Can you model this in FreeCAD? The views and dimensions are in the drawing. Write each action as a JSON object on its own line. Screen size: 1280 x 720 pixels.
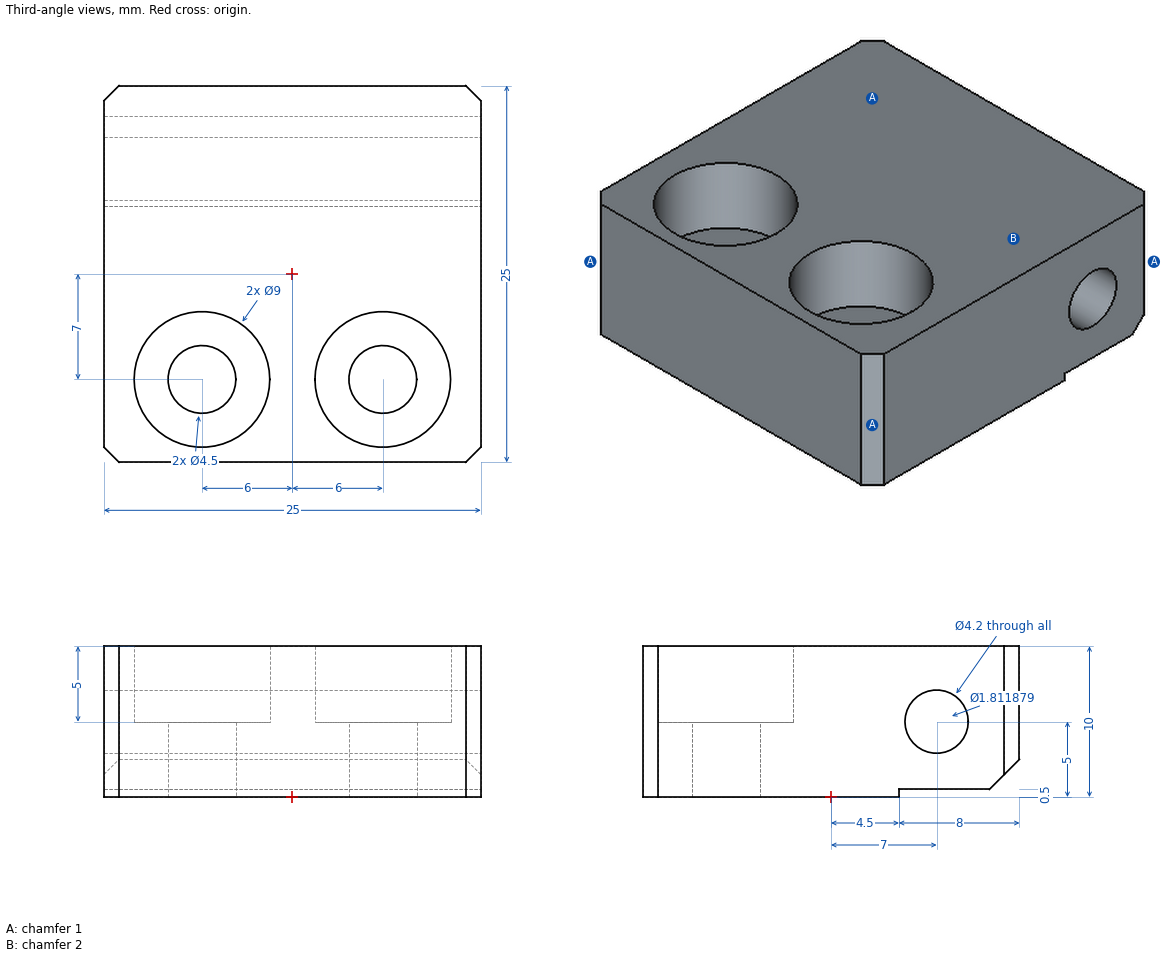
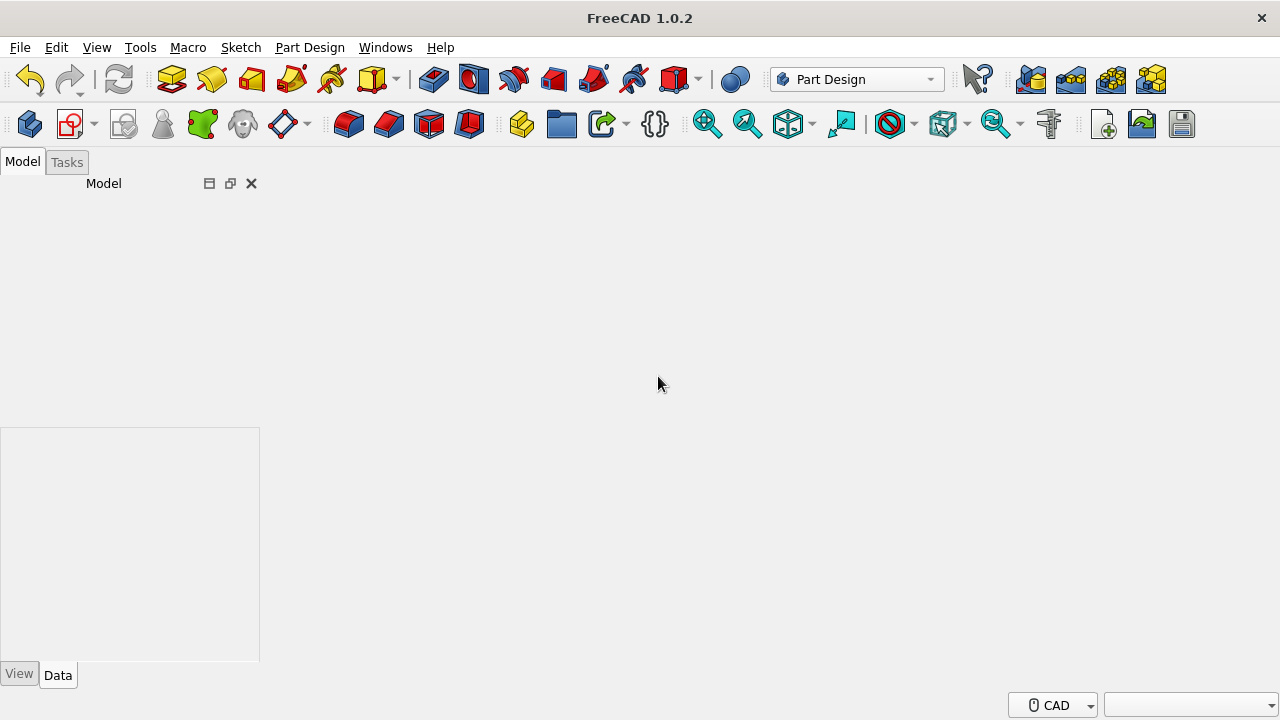
{"action": "key", "text": "ctrl+n"}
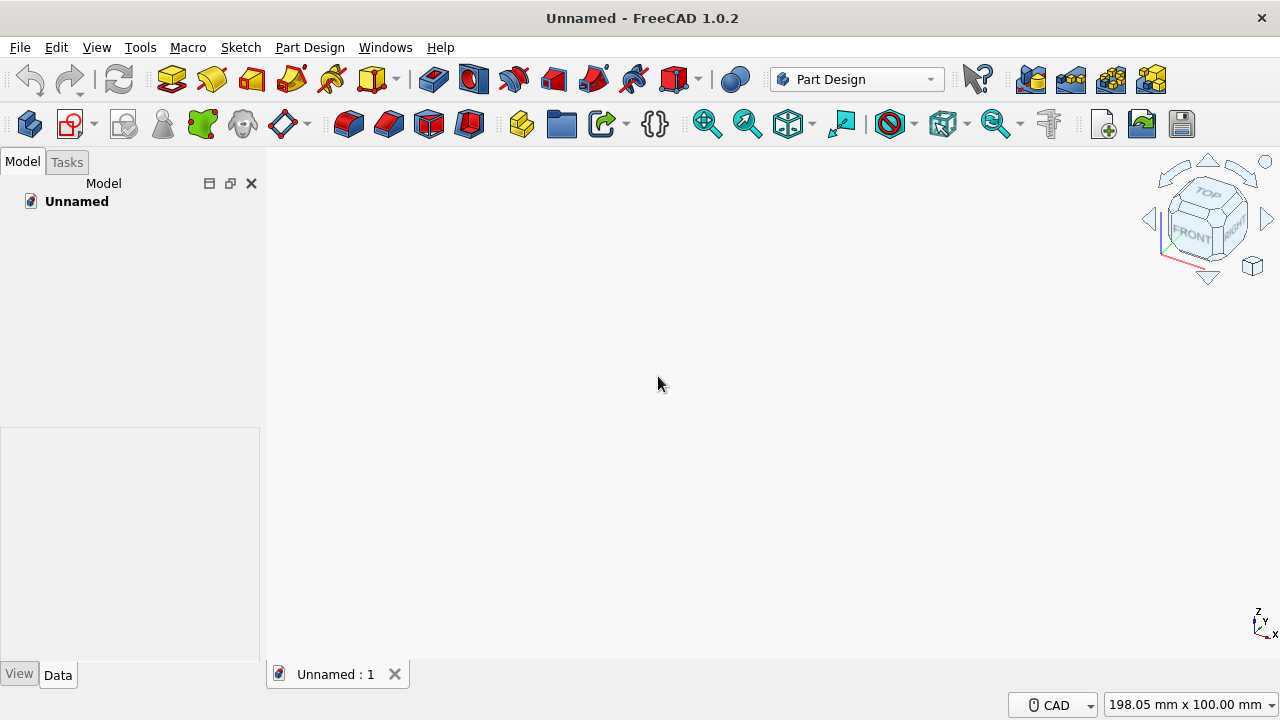
{"action": "left_click", "coordinate": [70, 124]}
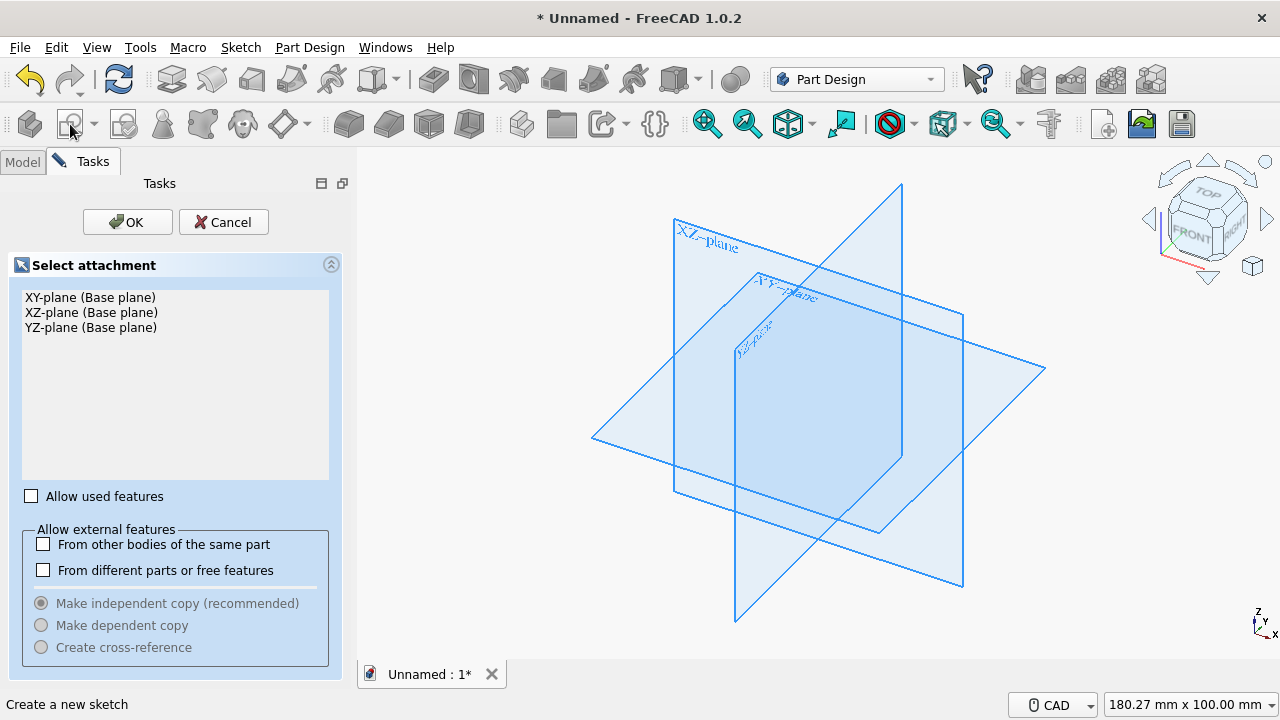
{"action": "left_click", "coordinate": [82, 298]}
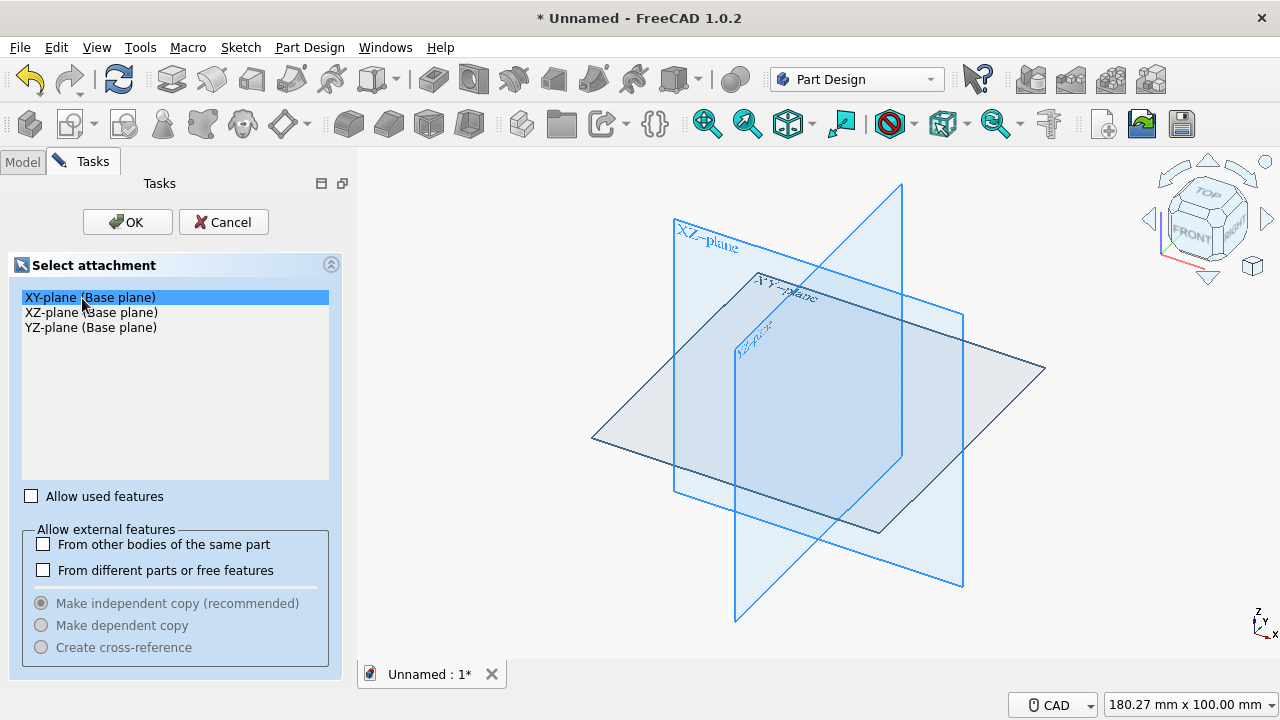
{"action": "left_click", "coordinate": [128, 222]}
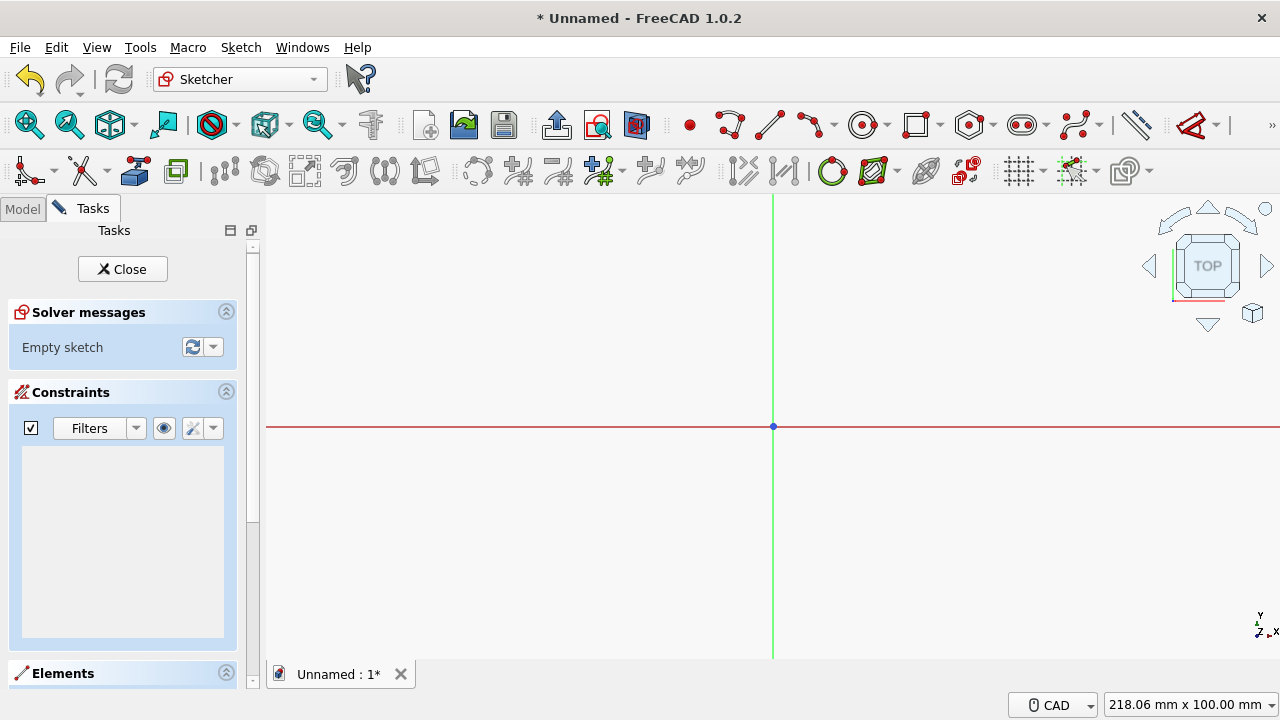
{"action": "scroll", "coordinate": [813, 426], "scroll_direction": "up", "scroll_amount": 5}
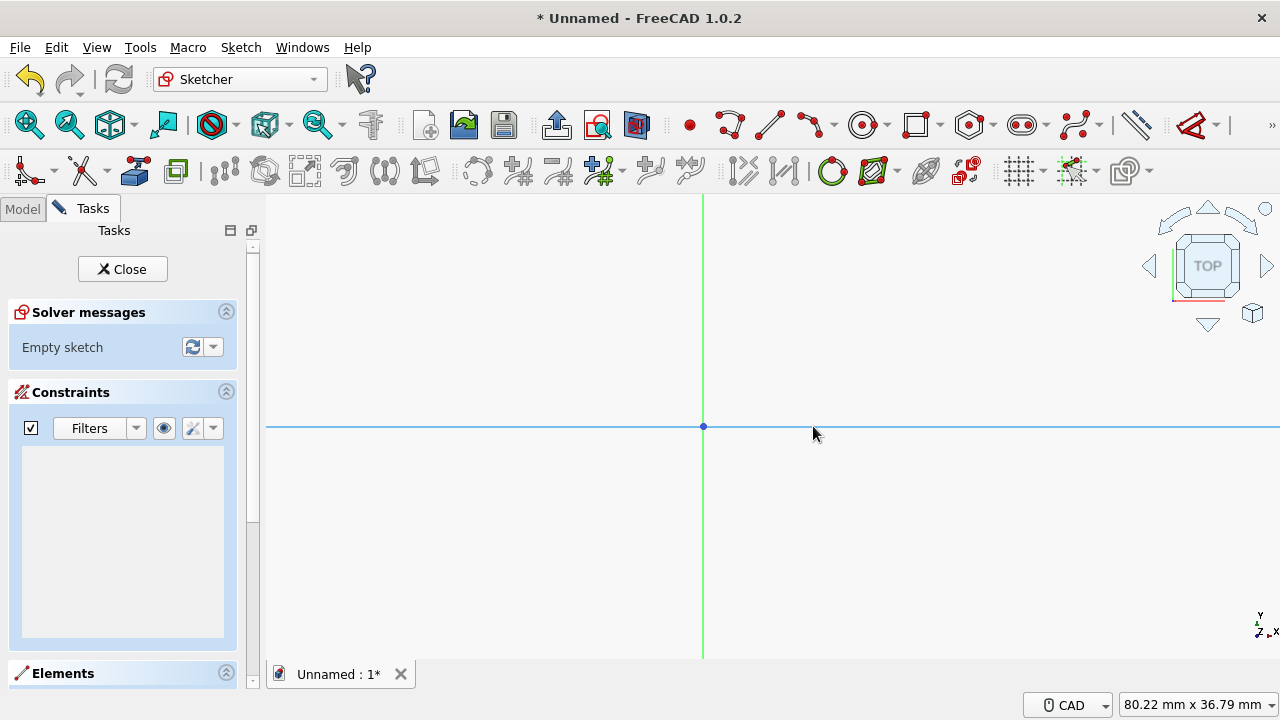
{"action": "key", "text": "g v"}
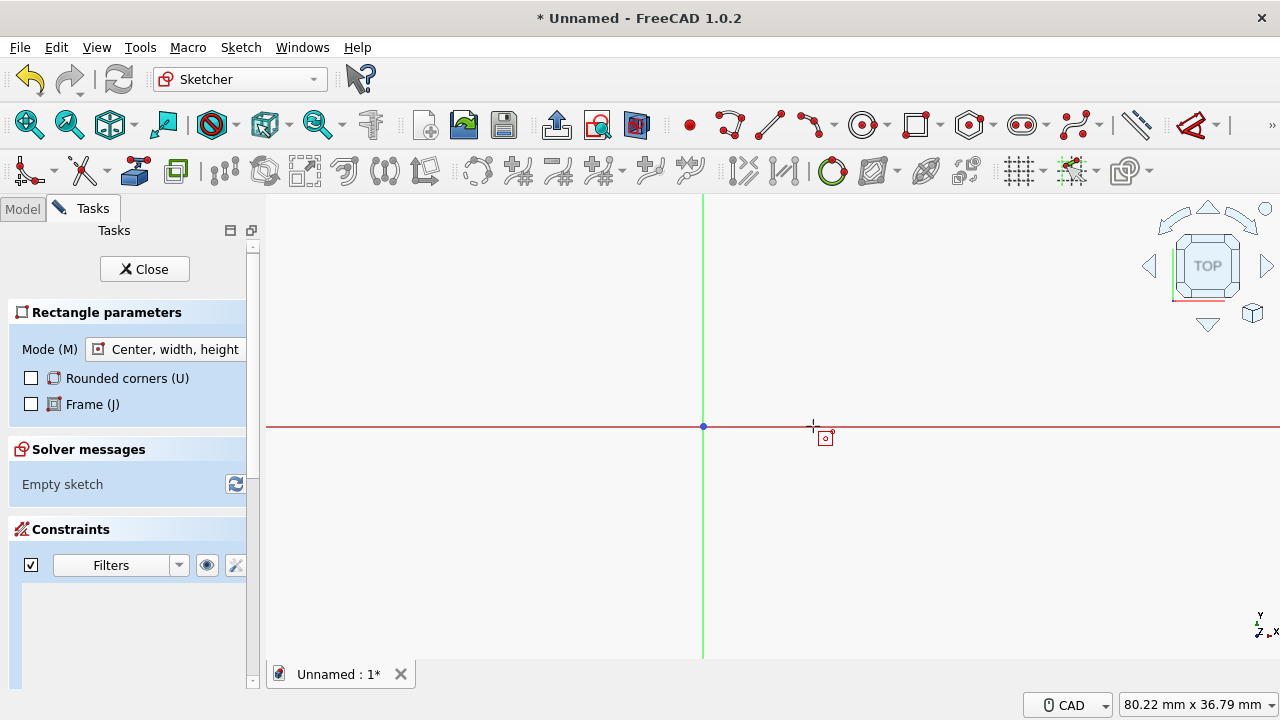
{"action": "left_click", "coordinate": [703, 426]}
{"action": "left_click", "coordinate": [861, 268]}
{"action": "key", "text": "Escape"}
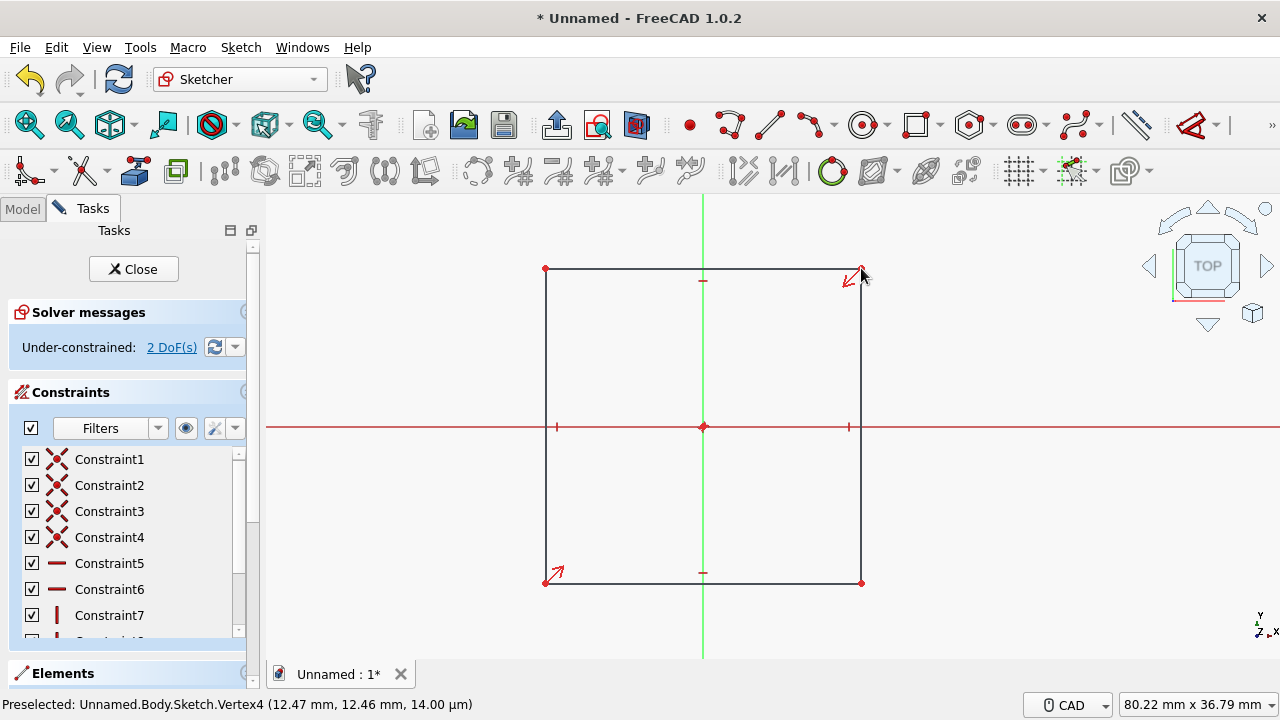
{"action": "key", "text": "d"}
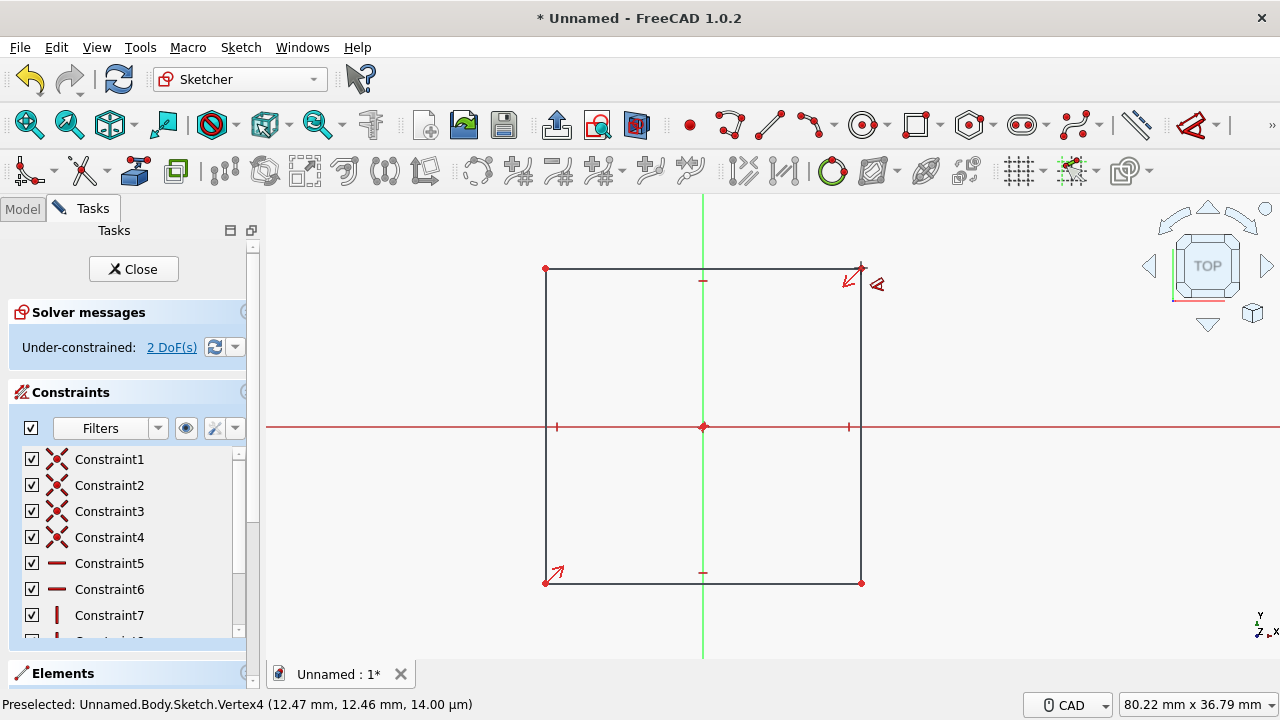
{"action": "left_click", "coordinate": [640, 584]}
{"action": "left_click", "coordinate": [631, 618]}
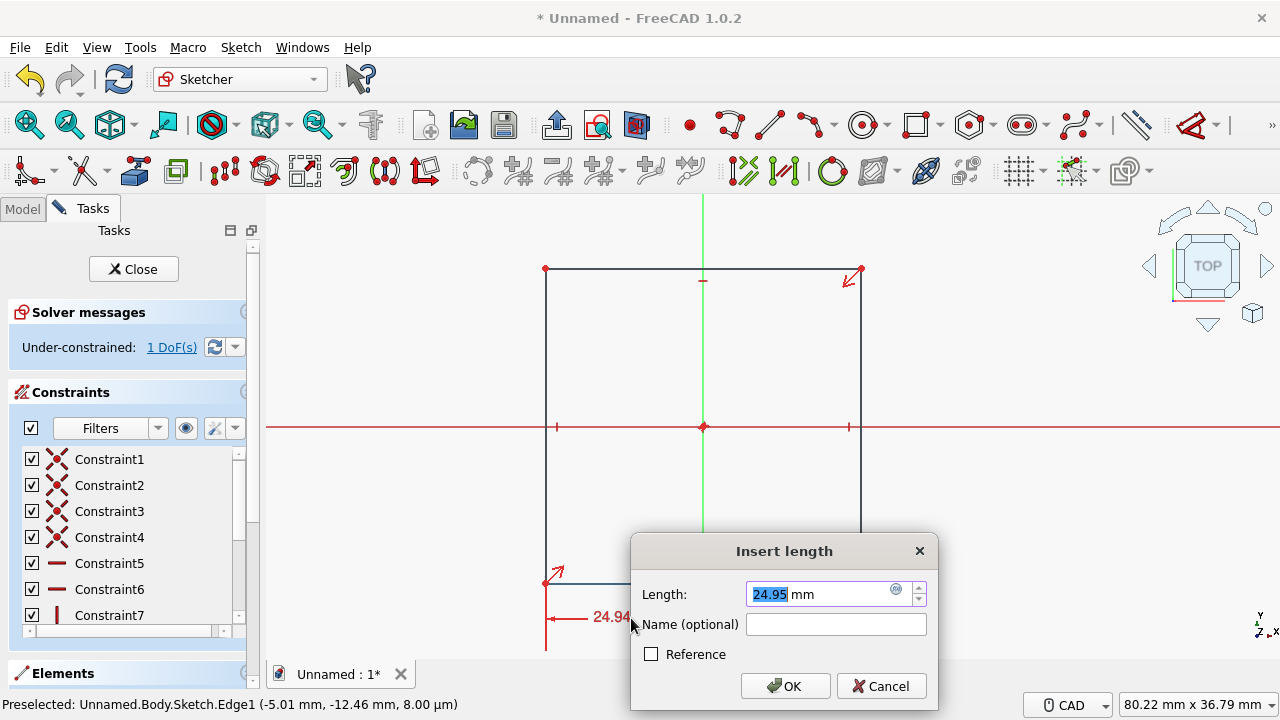
{"action": "type", "text": "25"}
{"action": "key", "text": "Return"}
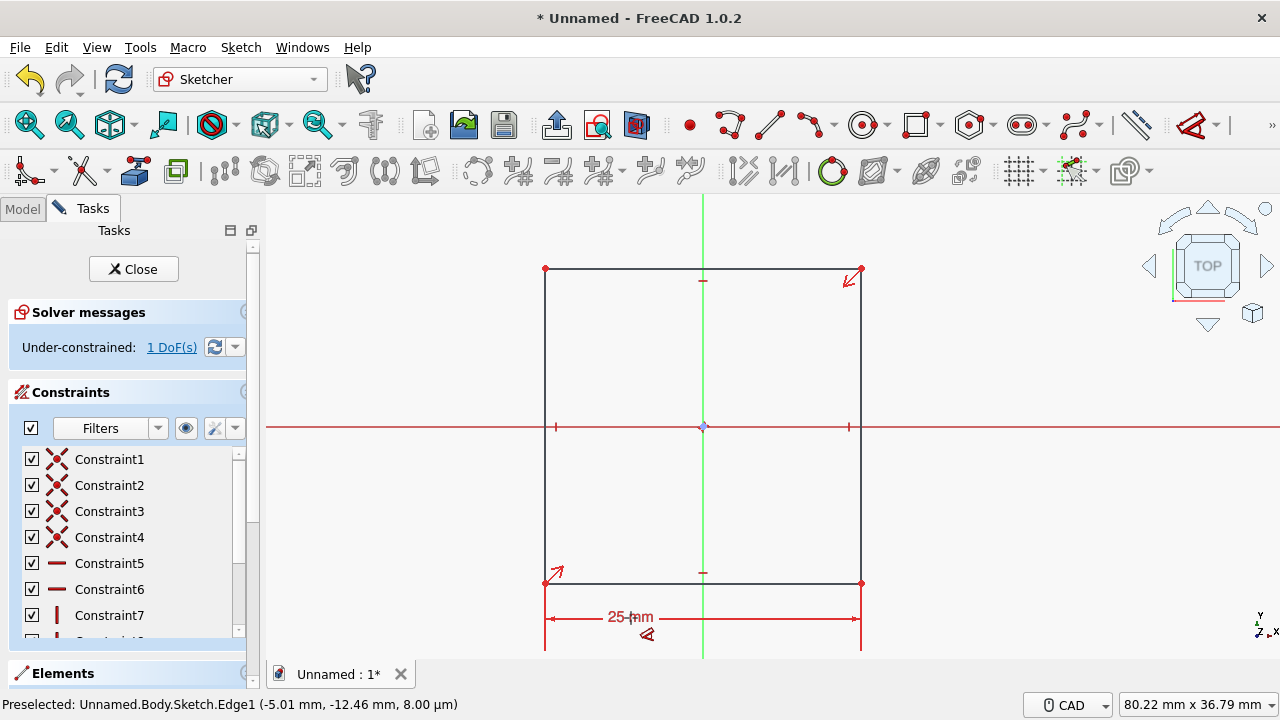
{"action": "left_click", "coordinate": [861, 489]}
{"action": "left_click", "coordinate": [895, 354]}